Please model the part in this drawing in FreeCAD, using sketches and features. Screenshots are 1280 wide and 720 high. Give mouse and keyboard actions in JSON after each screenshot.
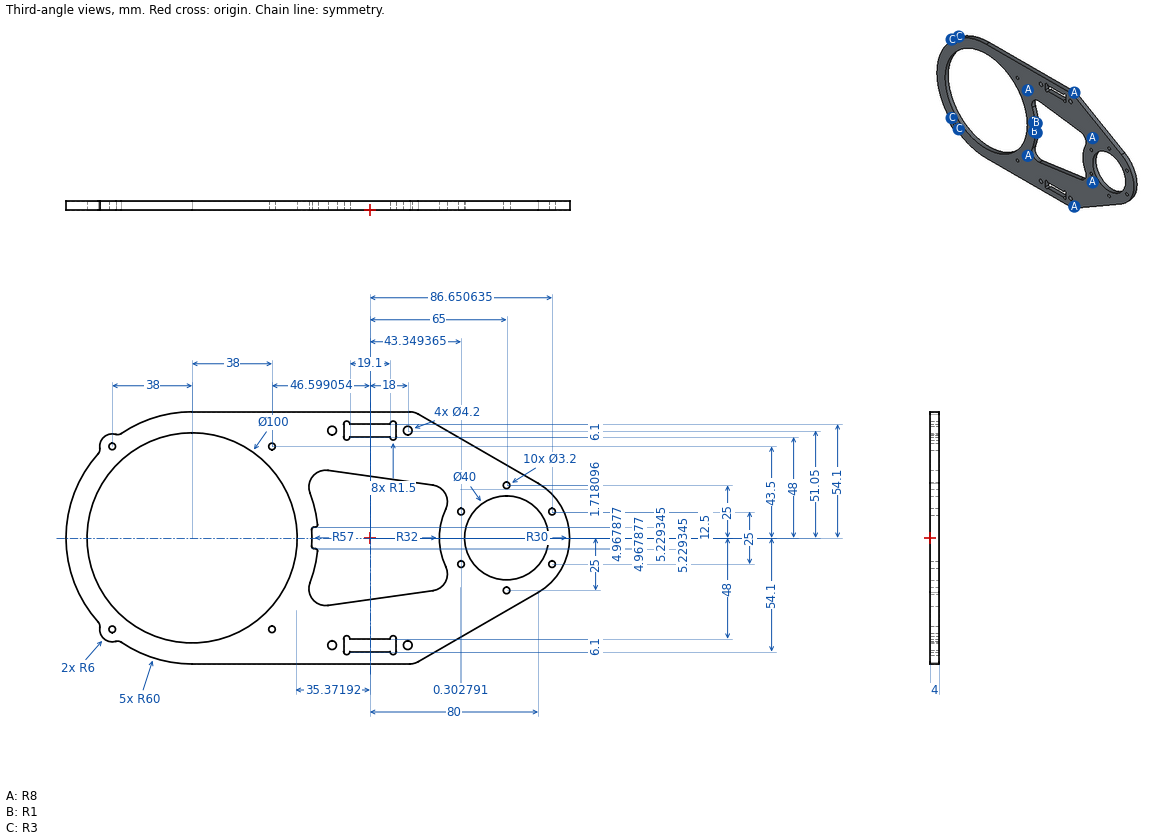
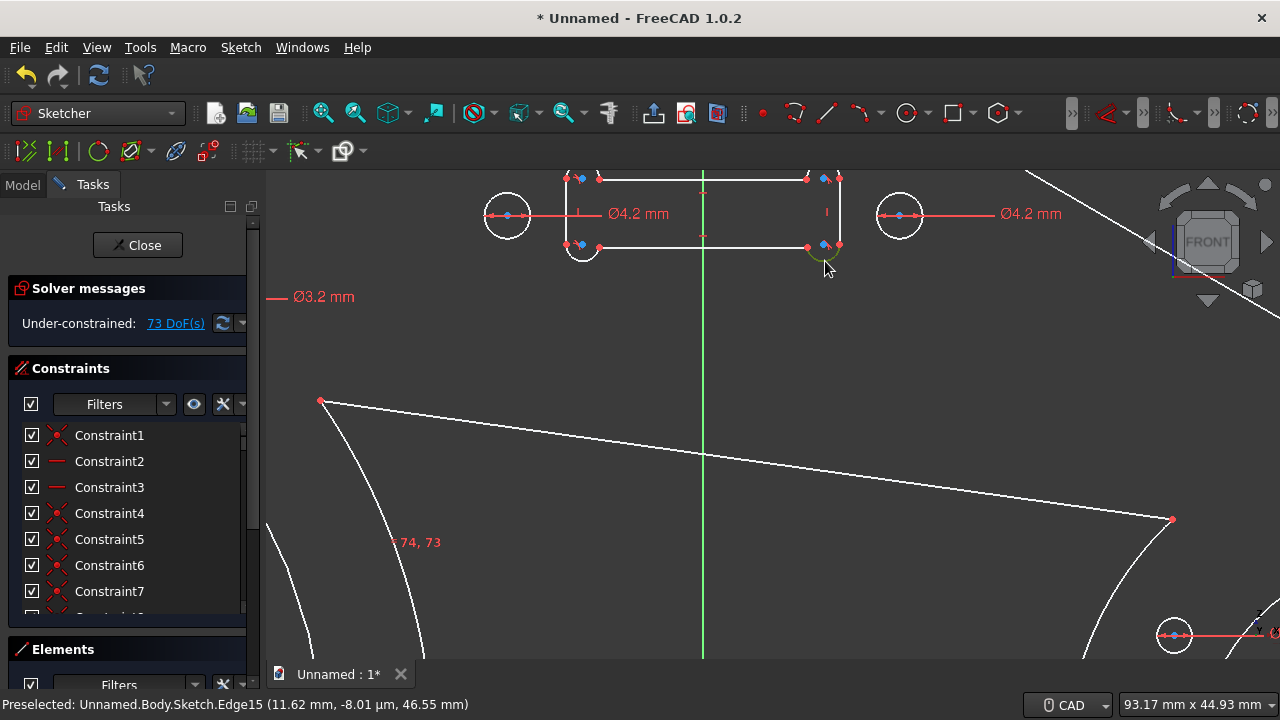
{"action": "scroll", "coordinate": [773, 325], "scroll_direction": "down", "scroll_amount": 8}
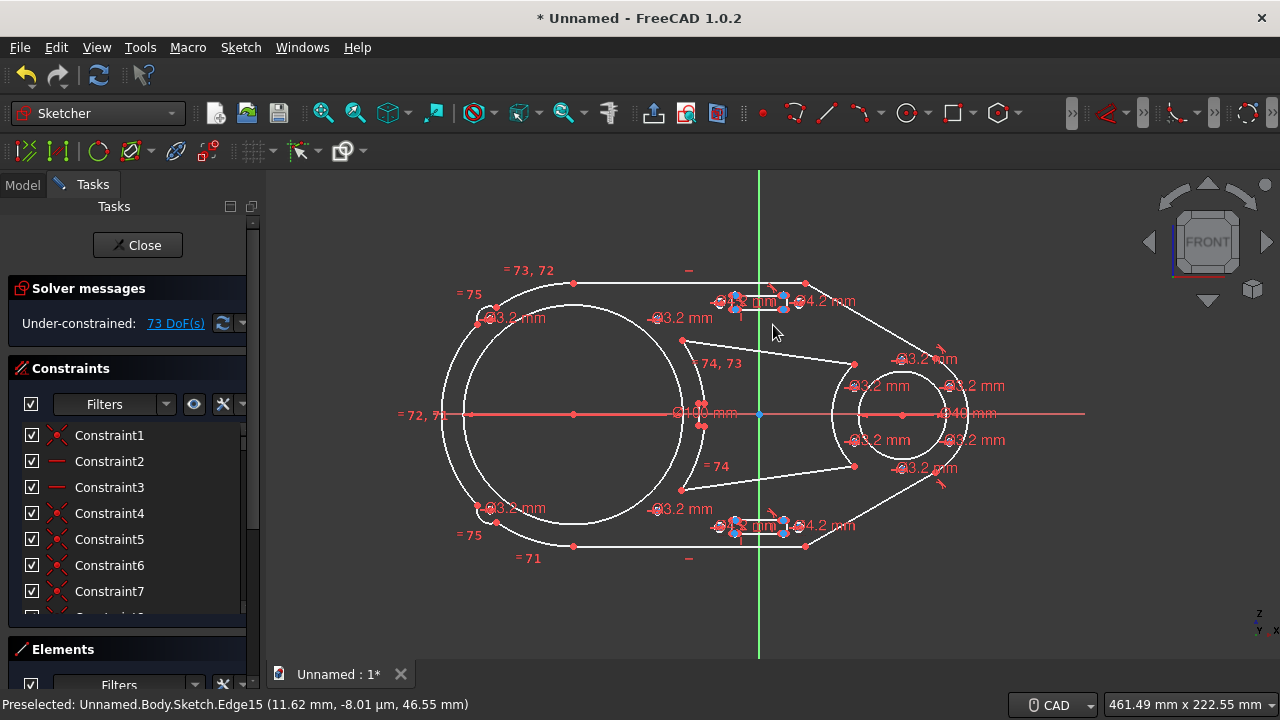
{"action": "scroll", "coordinate": [785, 293], "scroll_direction": "up", "scroll_amount": 8}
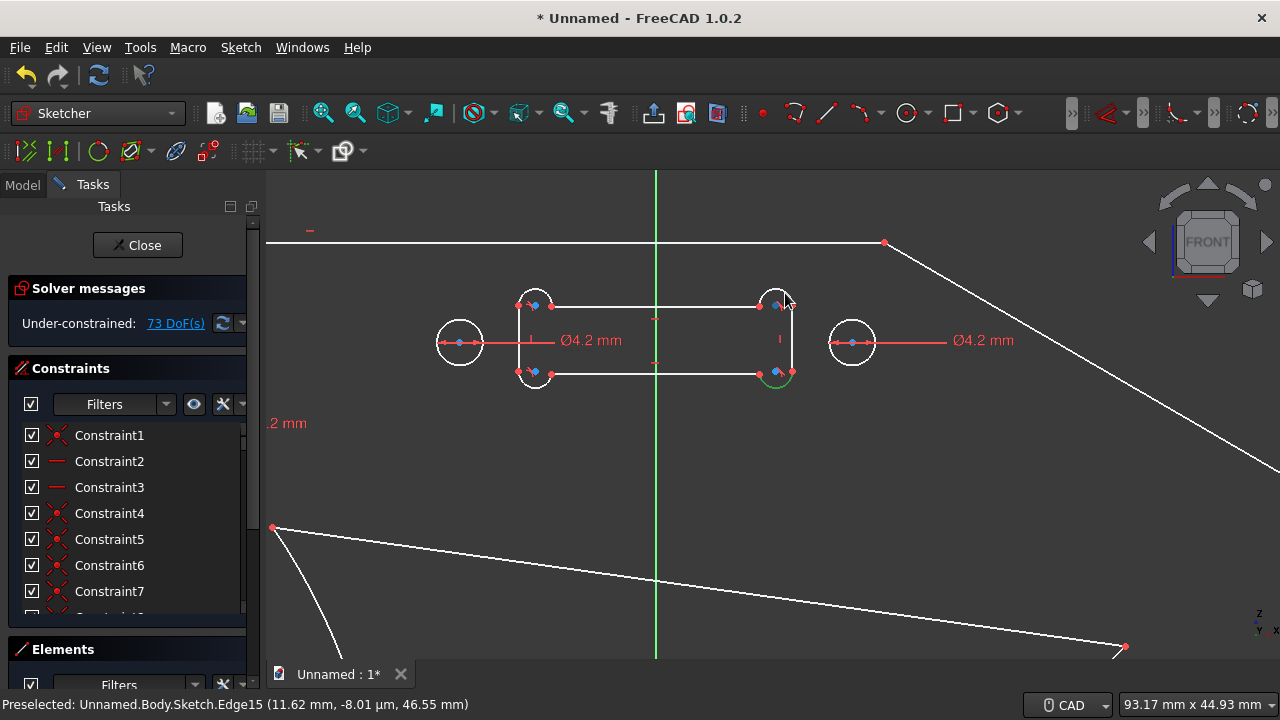
{"action": "left_click", "coordinate": [785, 292]}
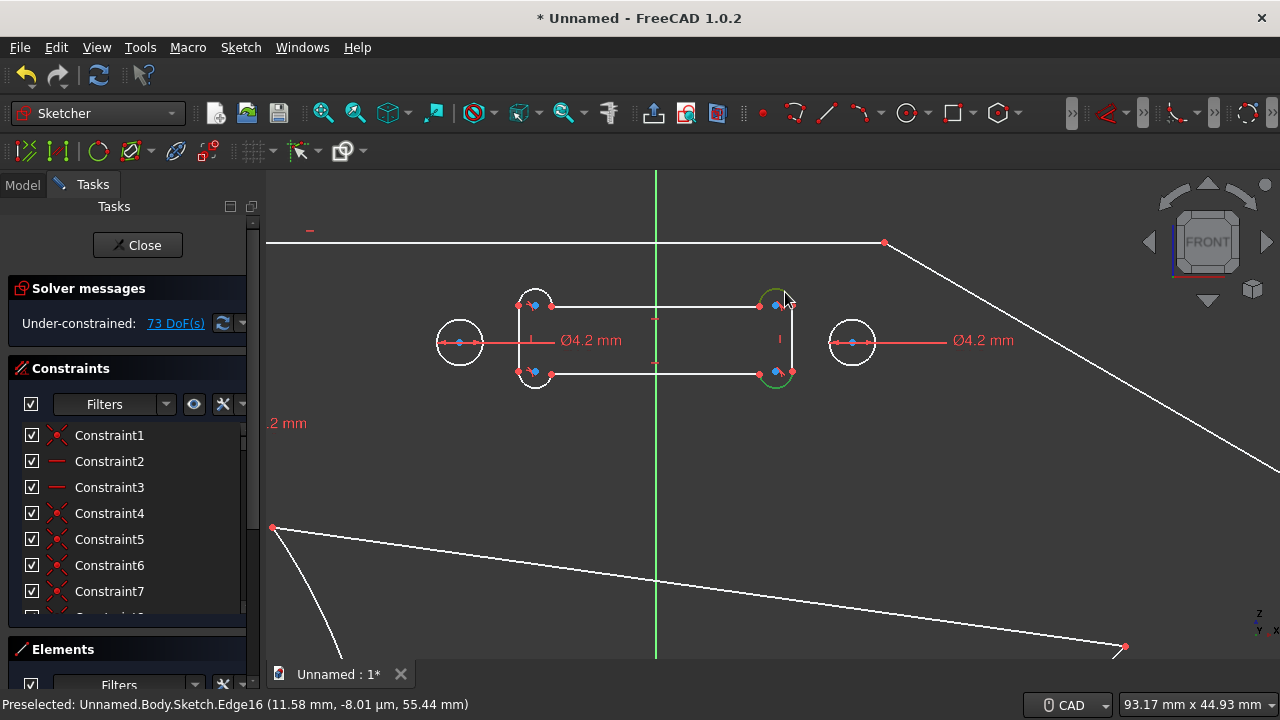
{"action": "left_click", "coordinate": [546, 293]}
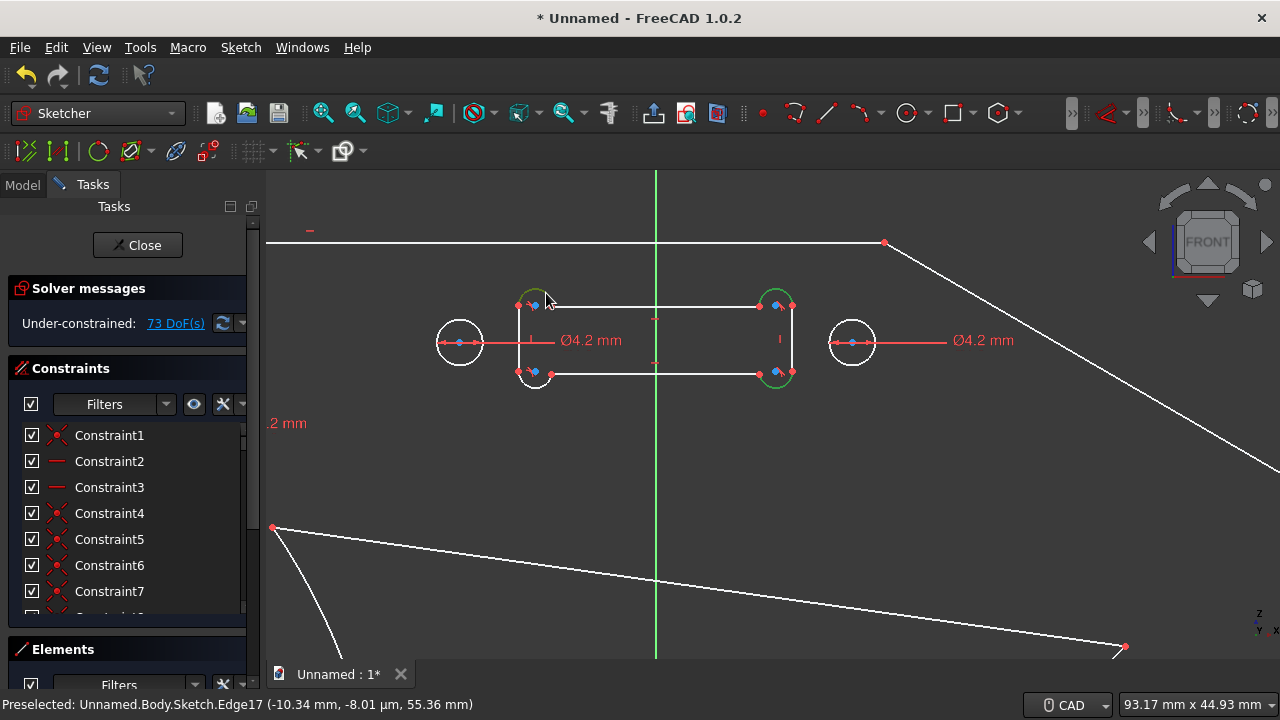
{"action": "left_click", "coordinate": [525, 384]}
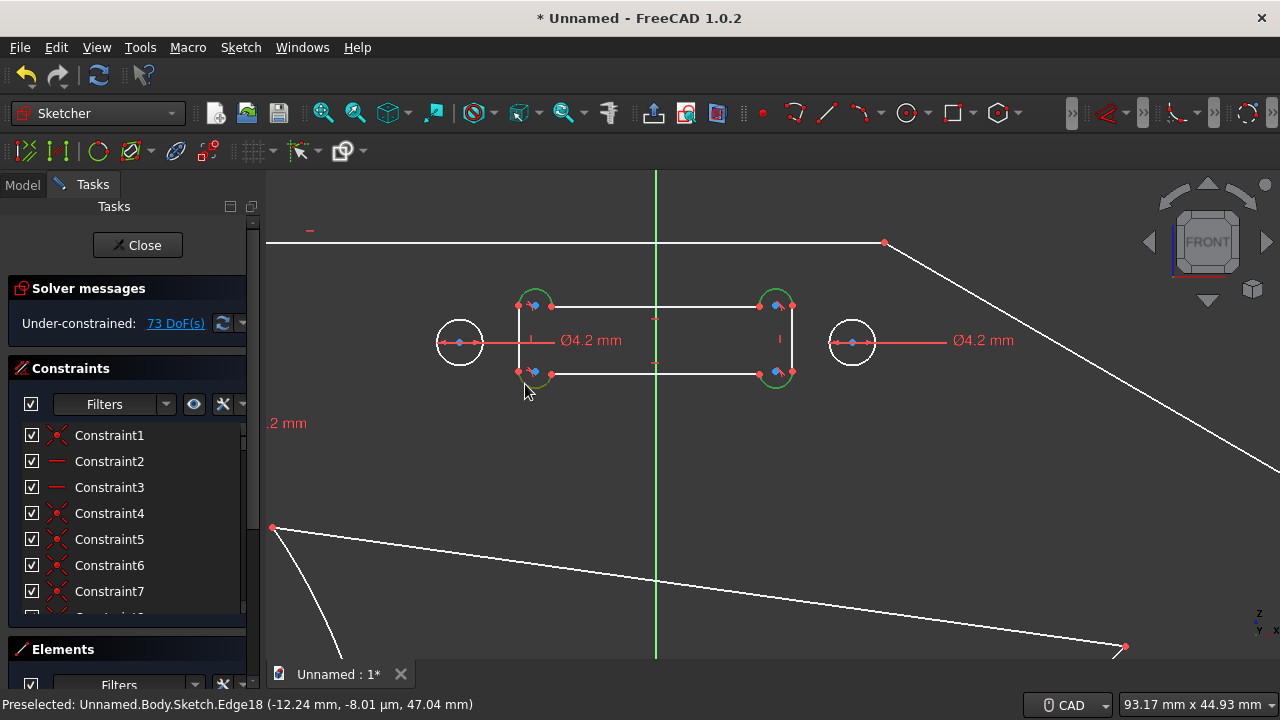
{"action": "scroll", "coordinate": [785, 293], "scroll_direction": "down", "scroll_amount": 8}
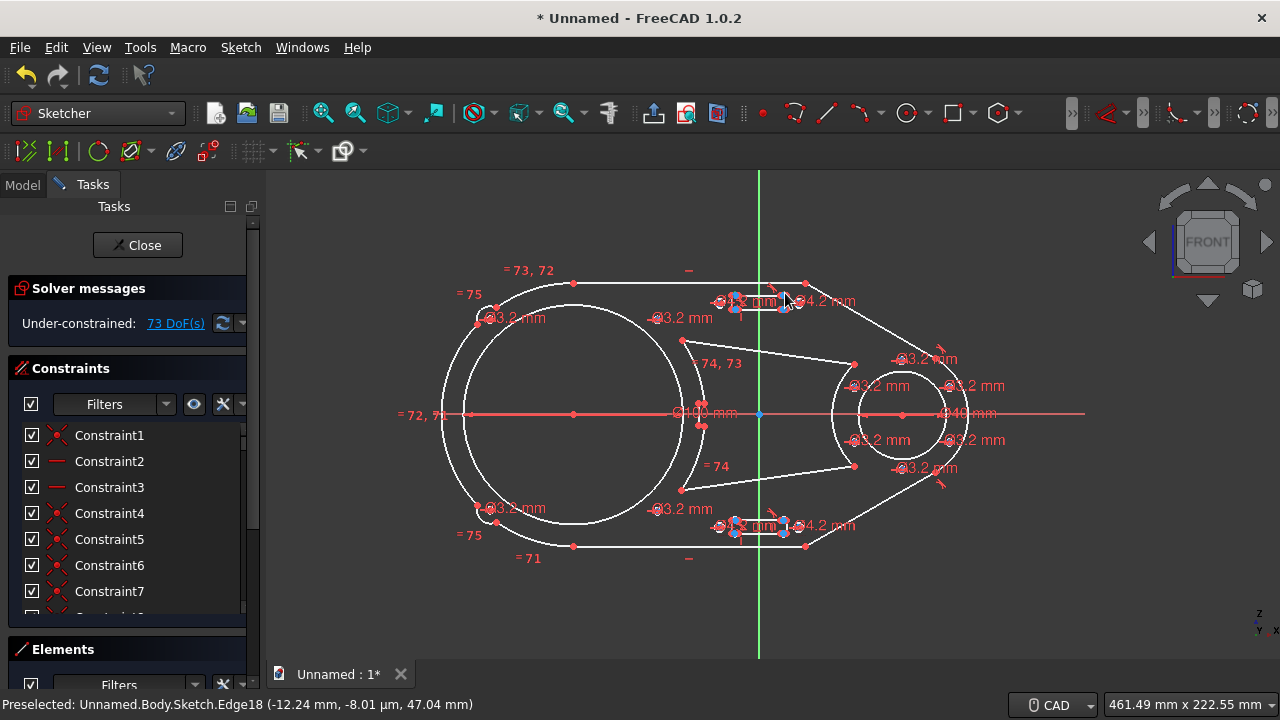
{"action": "scroll", "coordinate": [782, 536], "scroll_direction": "up", "scroll_amount": 8}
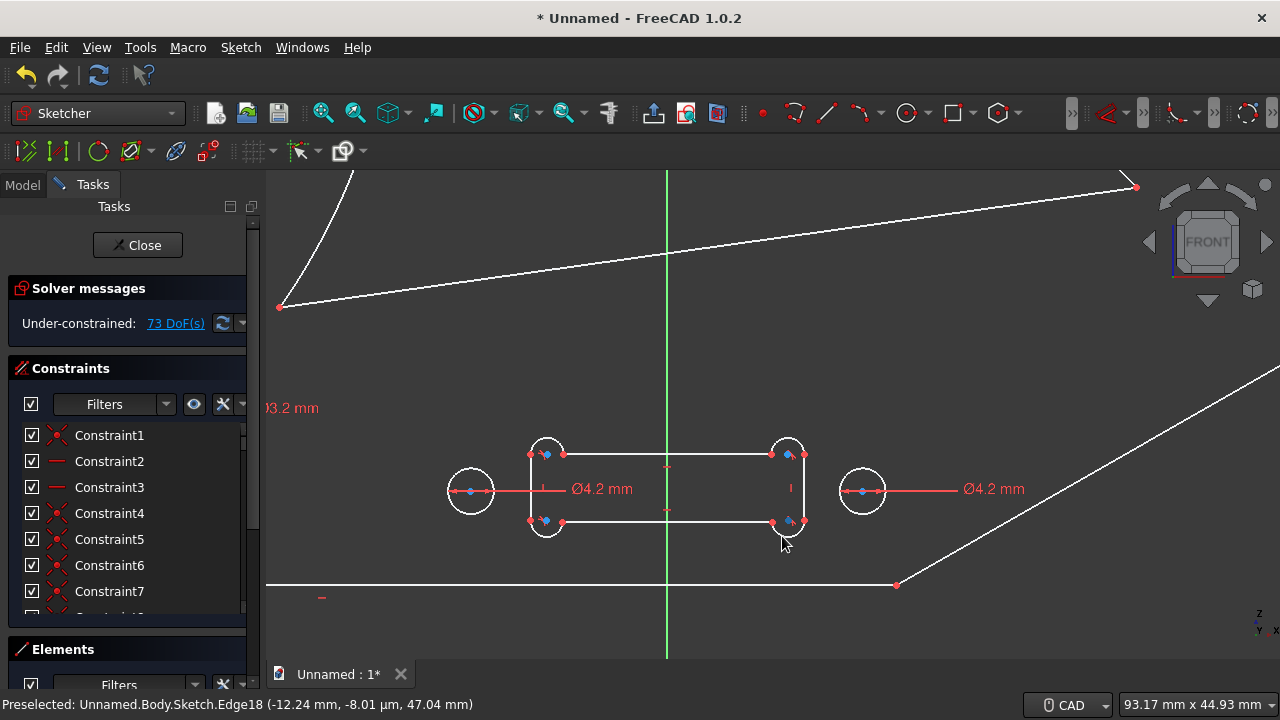
{"action": "left_click", "coordinate": [779, 534]}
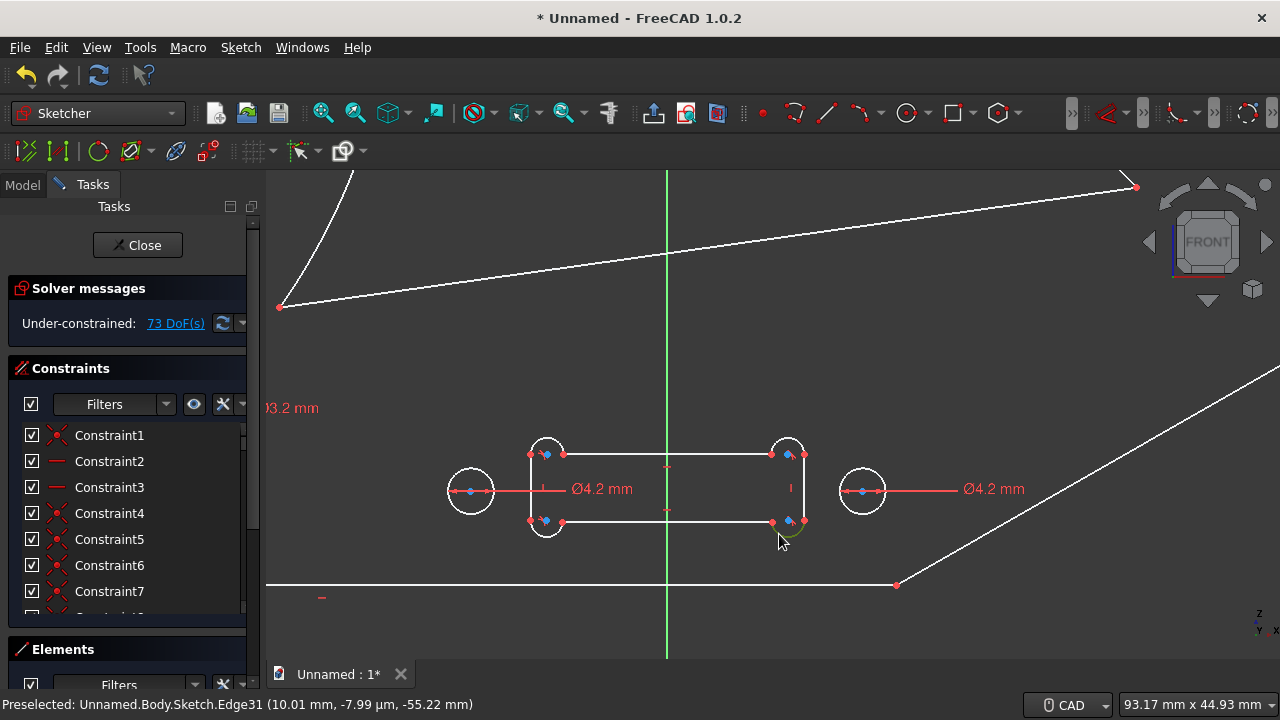
{"action": "left_click", "coordinate": [797, 441]}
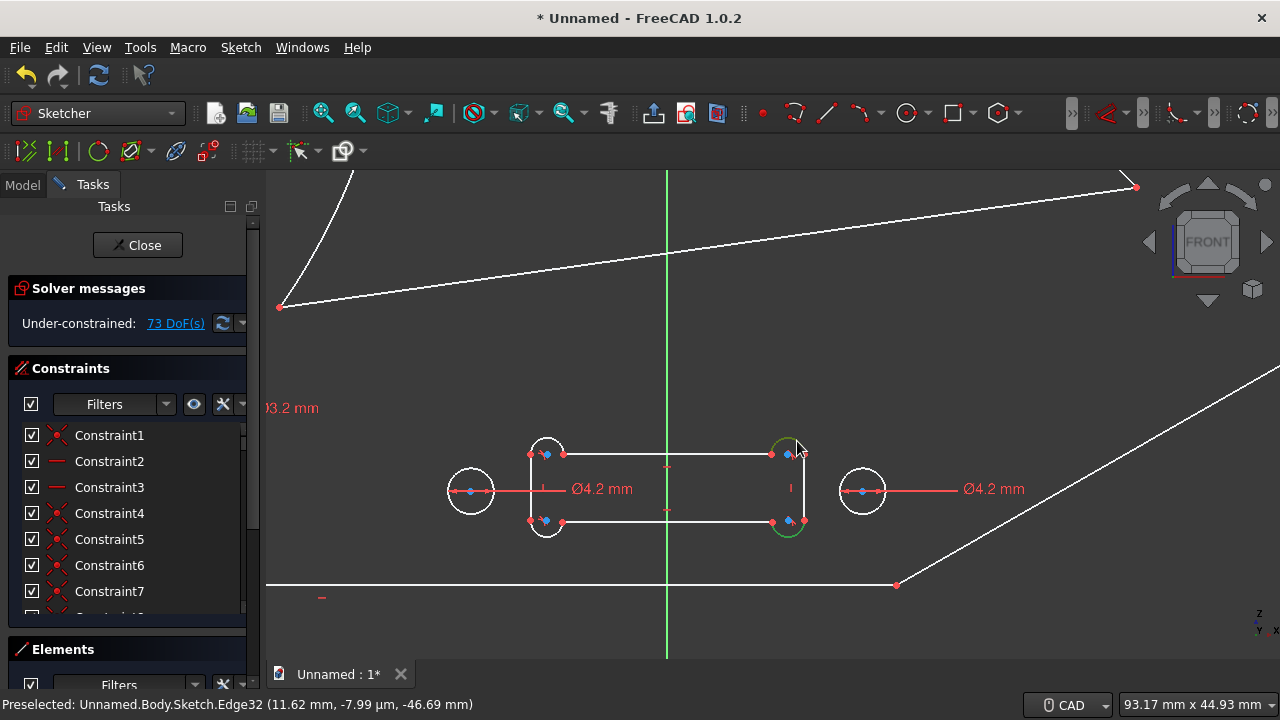
{"action": "left_click", "coordinate": [557, 441]}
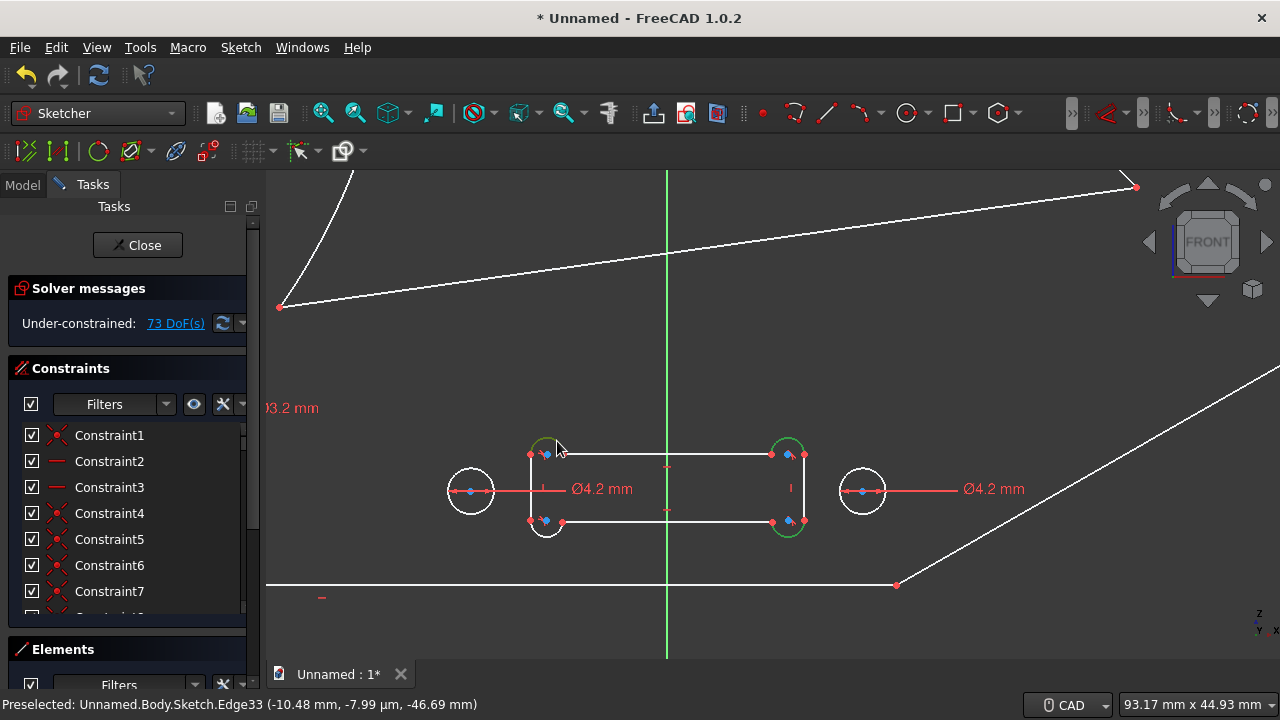
{"action": "left_click", "coordinate": [537, 534]}